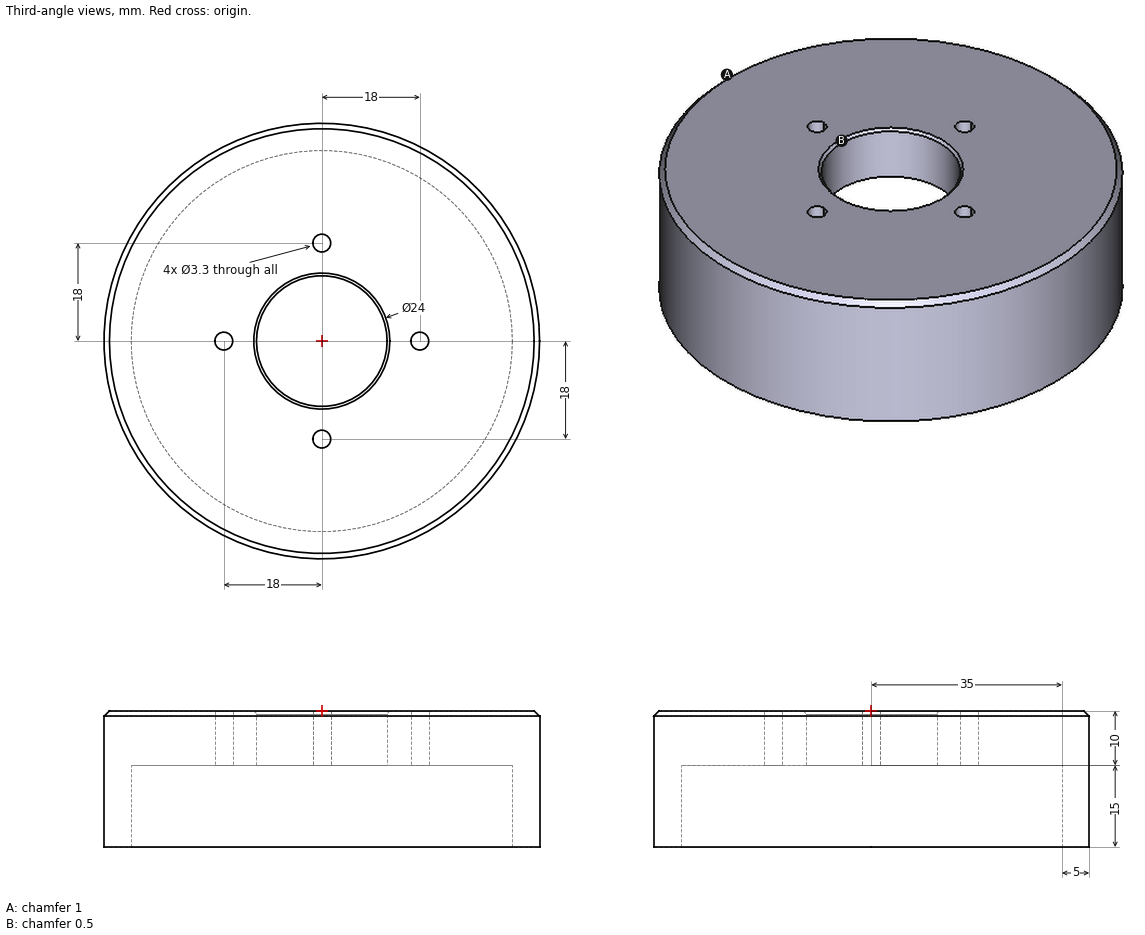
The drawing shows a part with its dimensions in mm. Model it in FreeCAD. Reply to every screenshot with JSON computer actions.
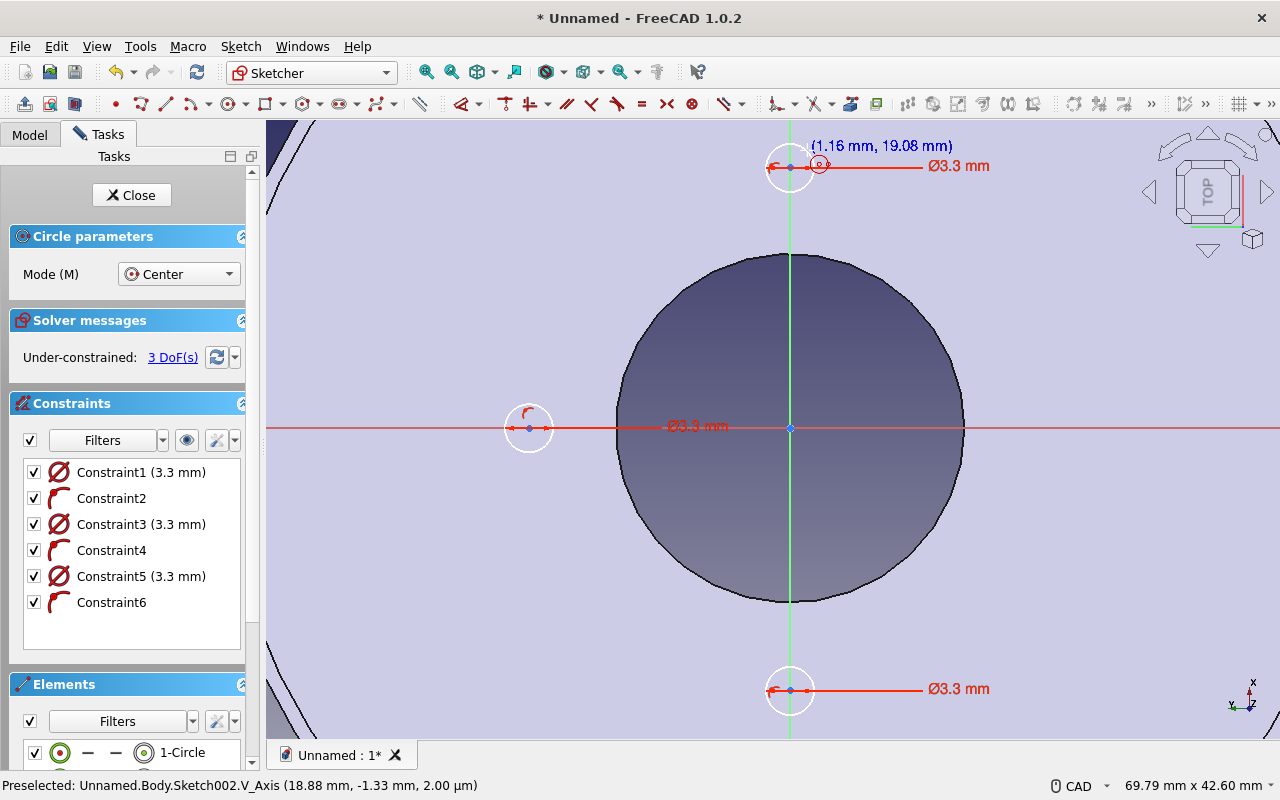
{"action": "left_click", "coordinate": [1052, 428]}
{"action": "mouse_move", "coordinate": [1069, 411]}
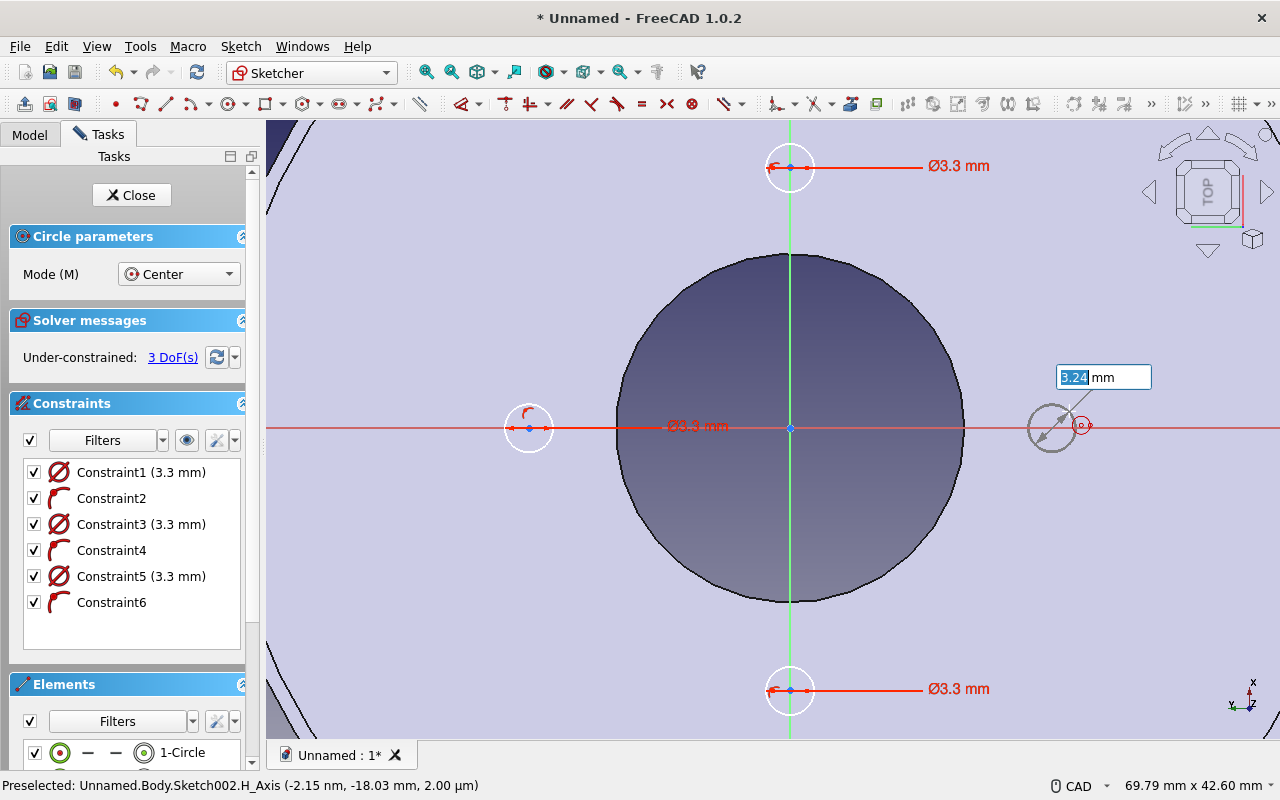
{"action": "type", "text": "3.3"}
{"action": "key", "text": "Return"}
{"action": "key", "text": "Escape"}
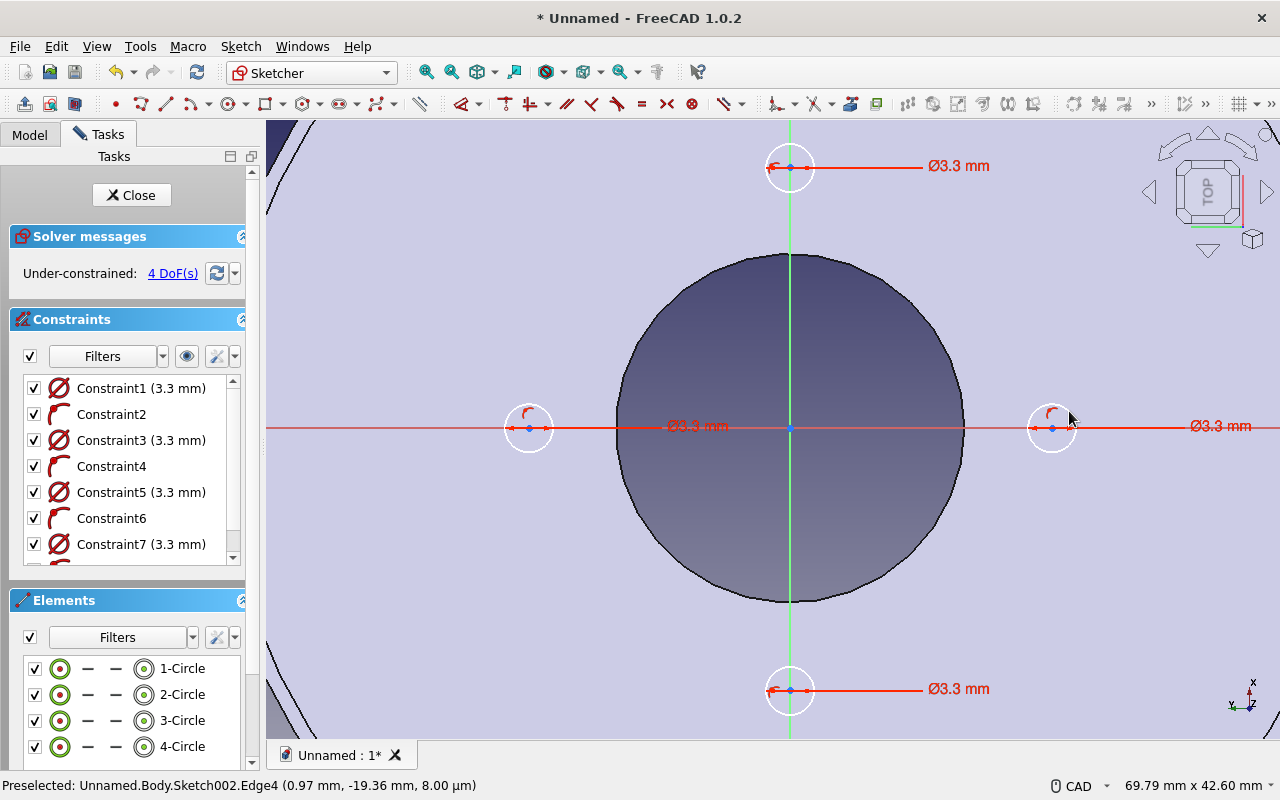
{"action": "key", "text": "d"}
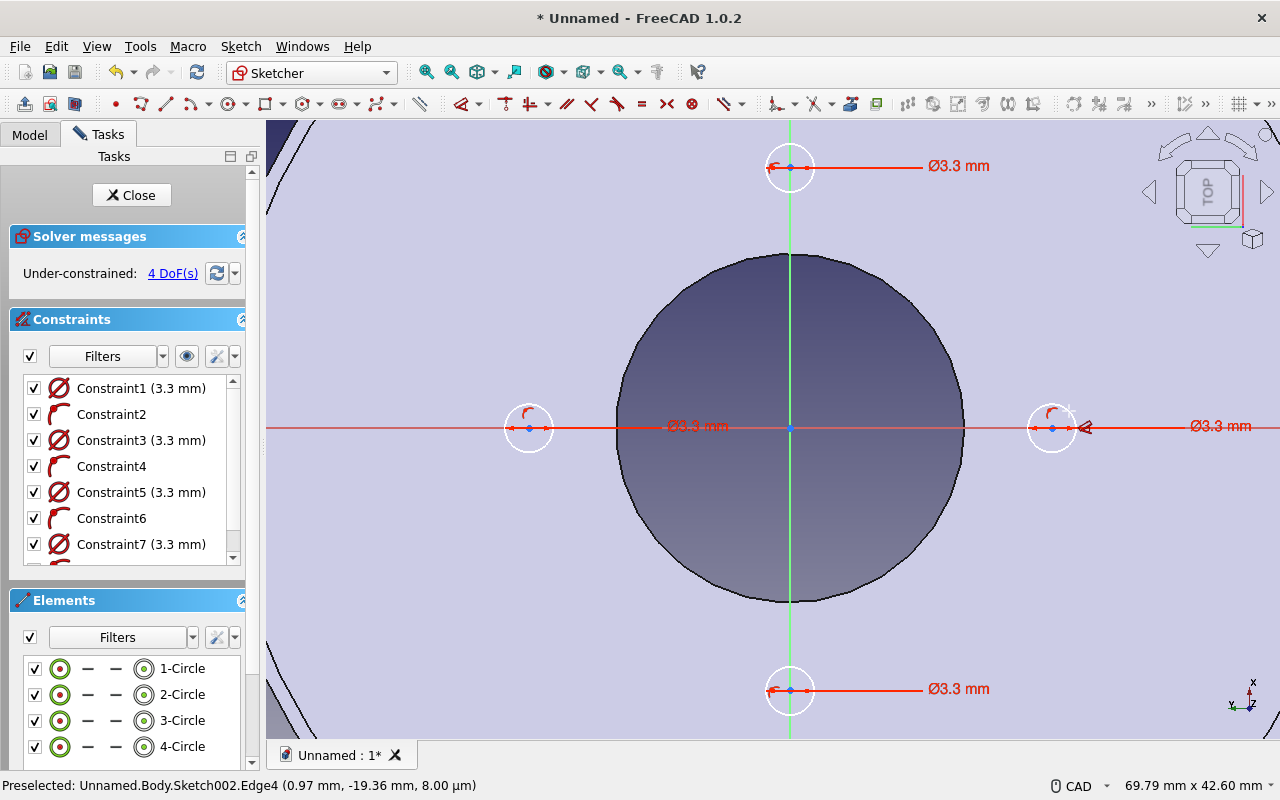
{"action": "left_click", "coordinate": [529, 428]}
{"action": "left_click", "coordinate": [660, 462]}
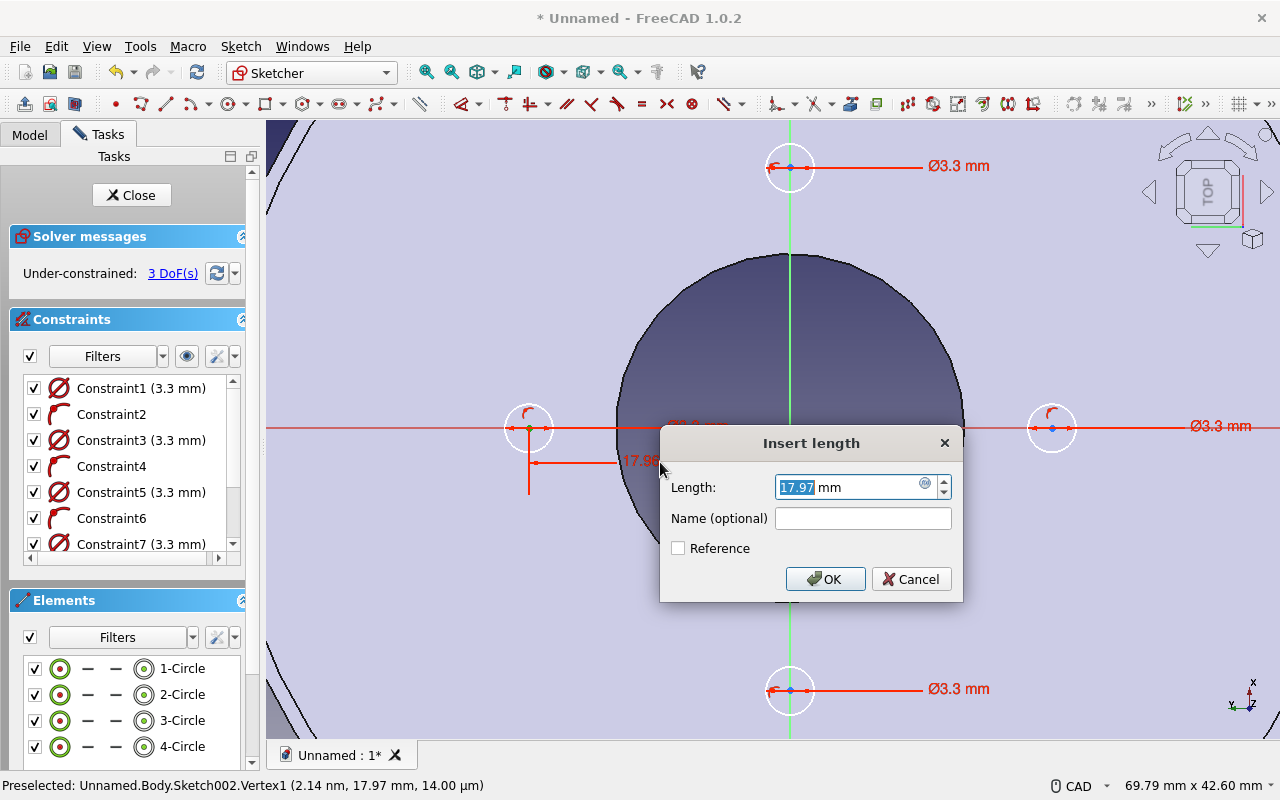
{"action": "type", "text": "18"}
{"action": "key", "text": "Return"}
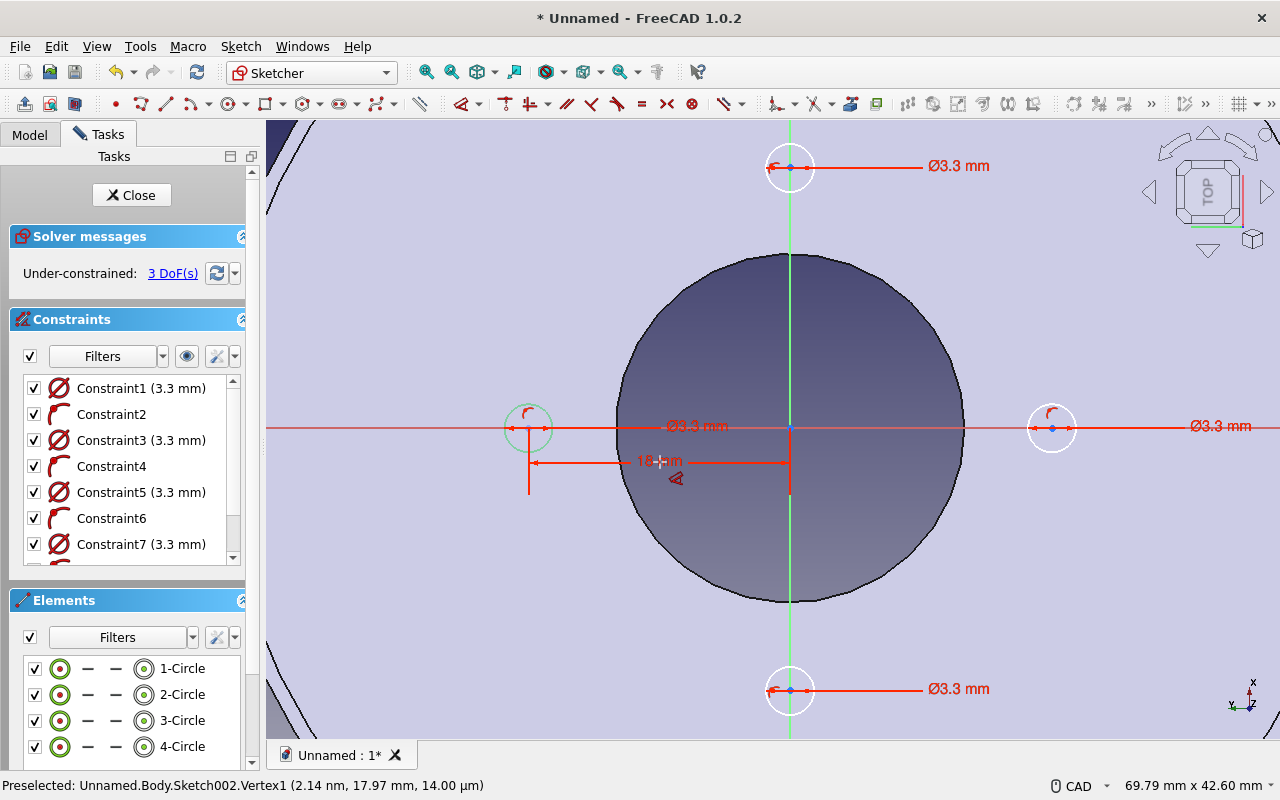
{"action": "left_click", "coordinate": [790, 691]}
{"action": "left_click", "coordinate": [824, 560]}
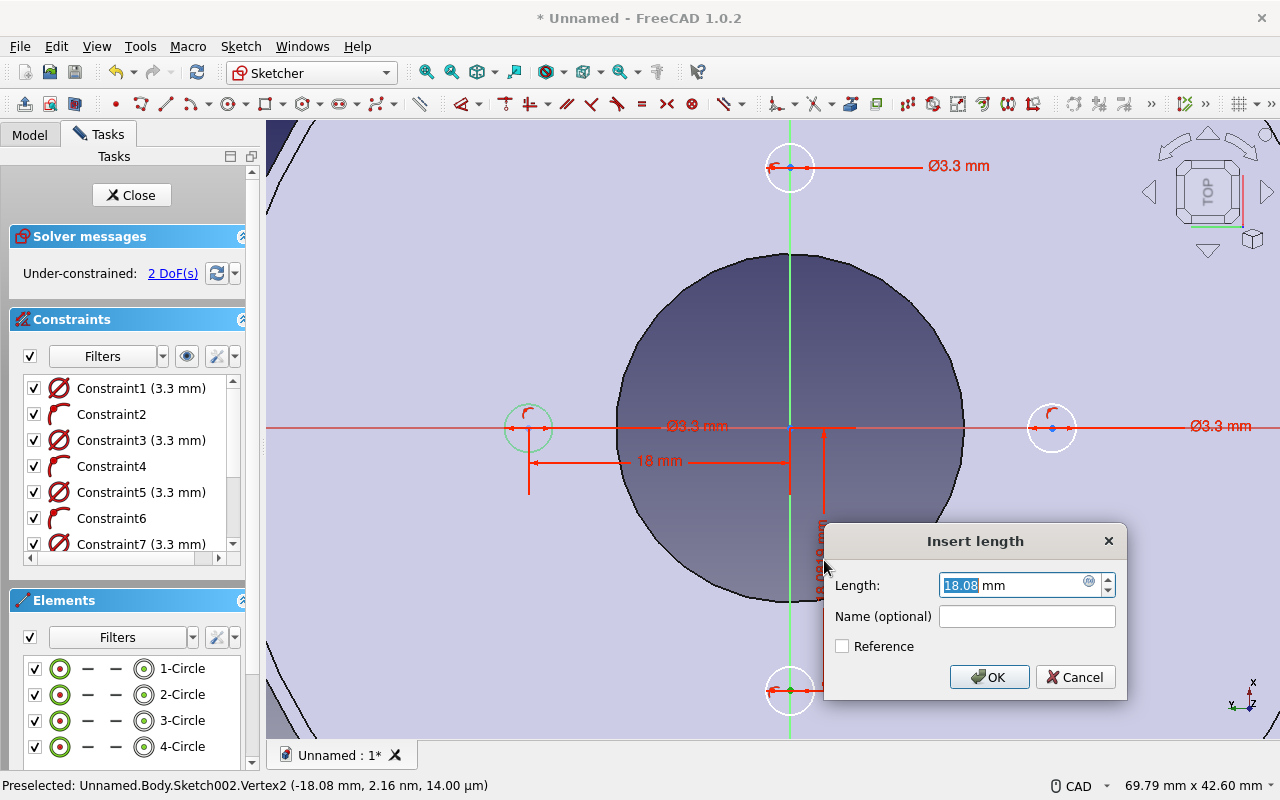
{"action": "type", "text": "18"}
{"action": "key", "text": "Return"}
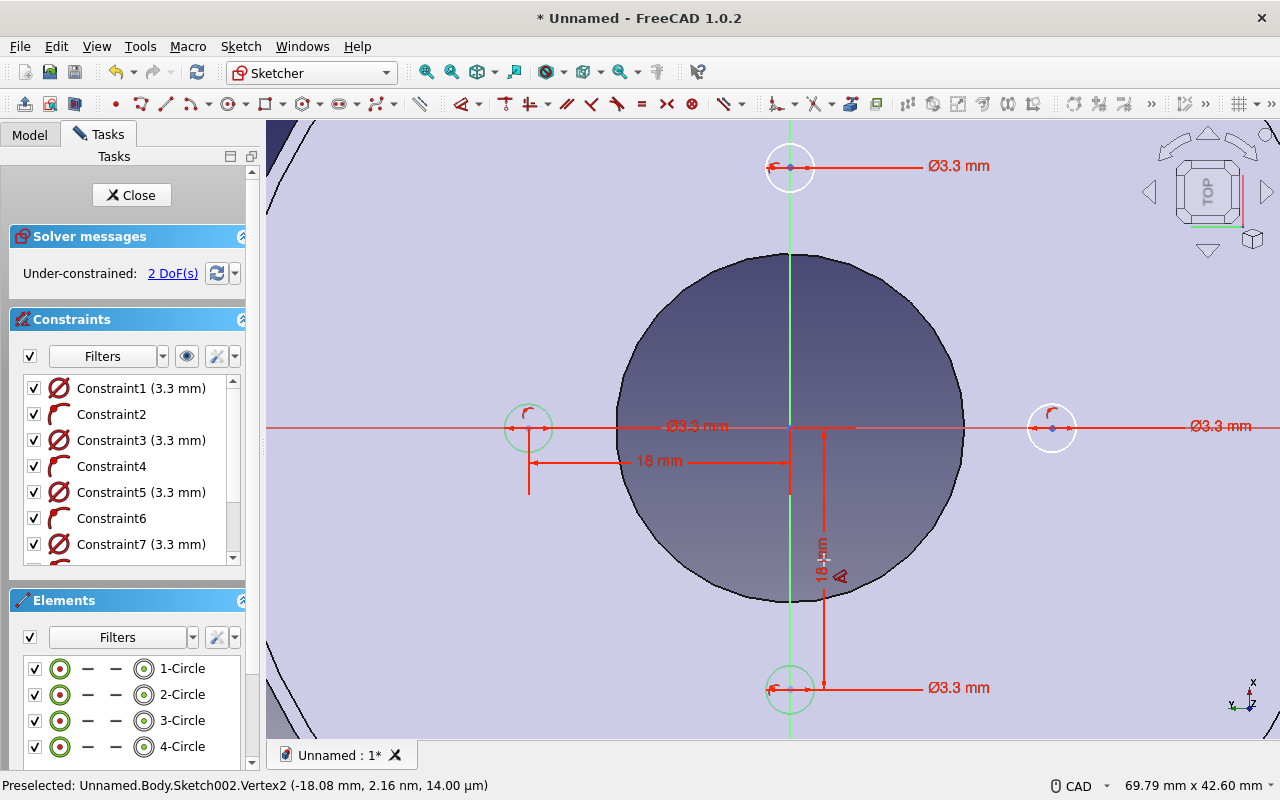
{"action": "left_click", "coordinate": [790, 168]}
{"action": "left_click", "coordinate": [824, 298]}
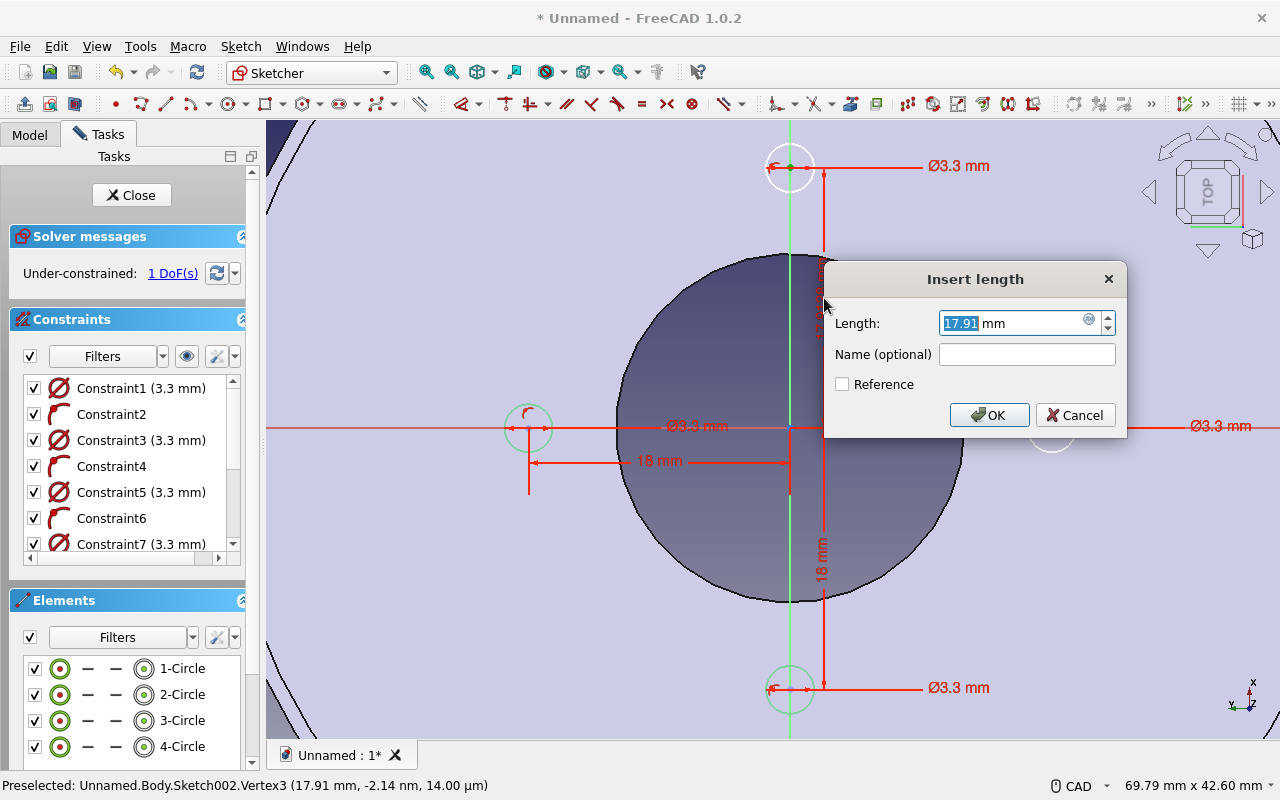
{"action": "type", "text": "18"}
{"action": "key", "text": "Return"}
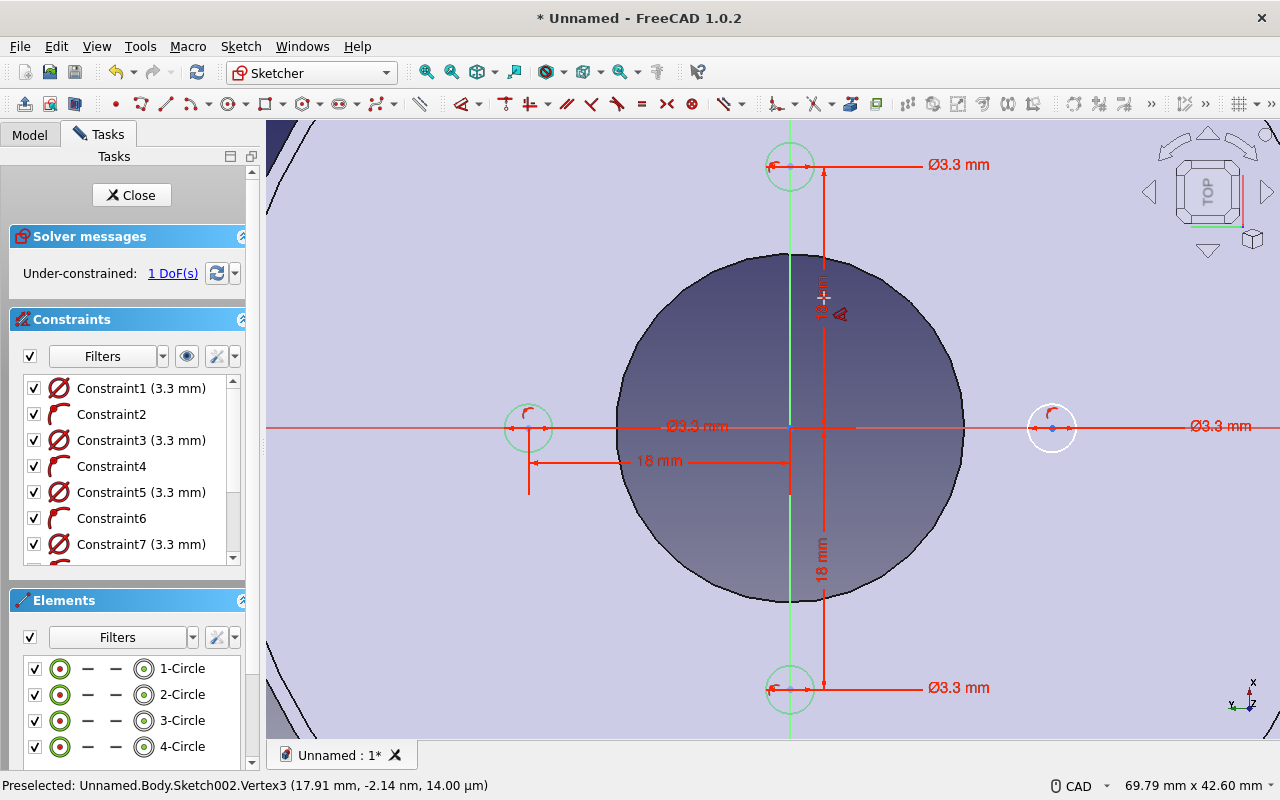
{"action": "left_click", "coordinate": [1052, 428]}
{"action": "left_click", "coordinate": [921, 394]}